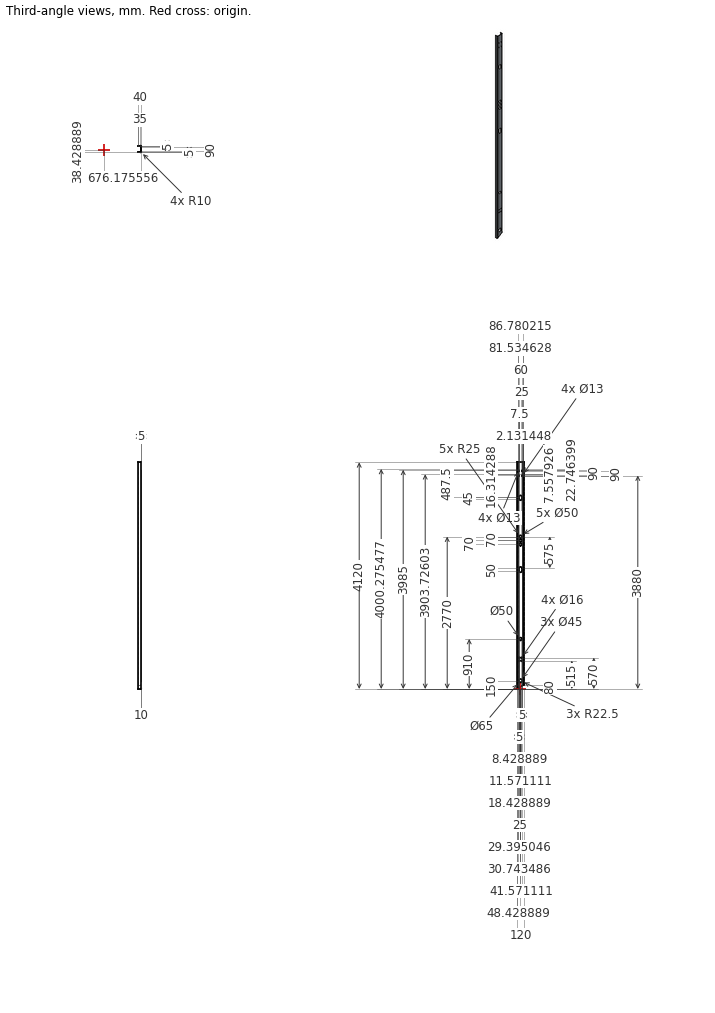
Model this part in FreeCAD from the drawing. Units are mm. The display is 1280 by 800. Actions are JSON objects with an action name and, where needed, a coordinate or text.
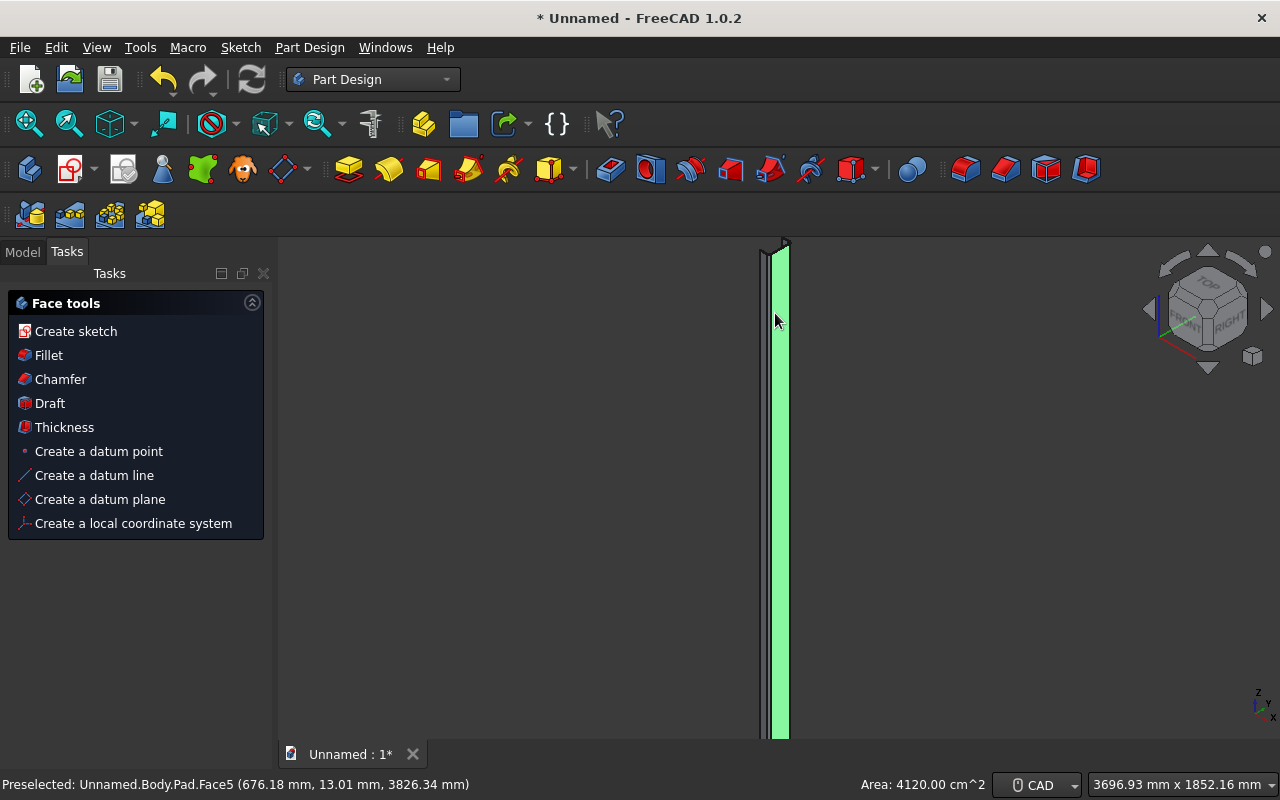
{"action": "left_click", "coordinate": [70, 170]}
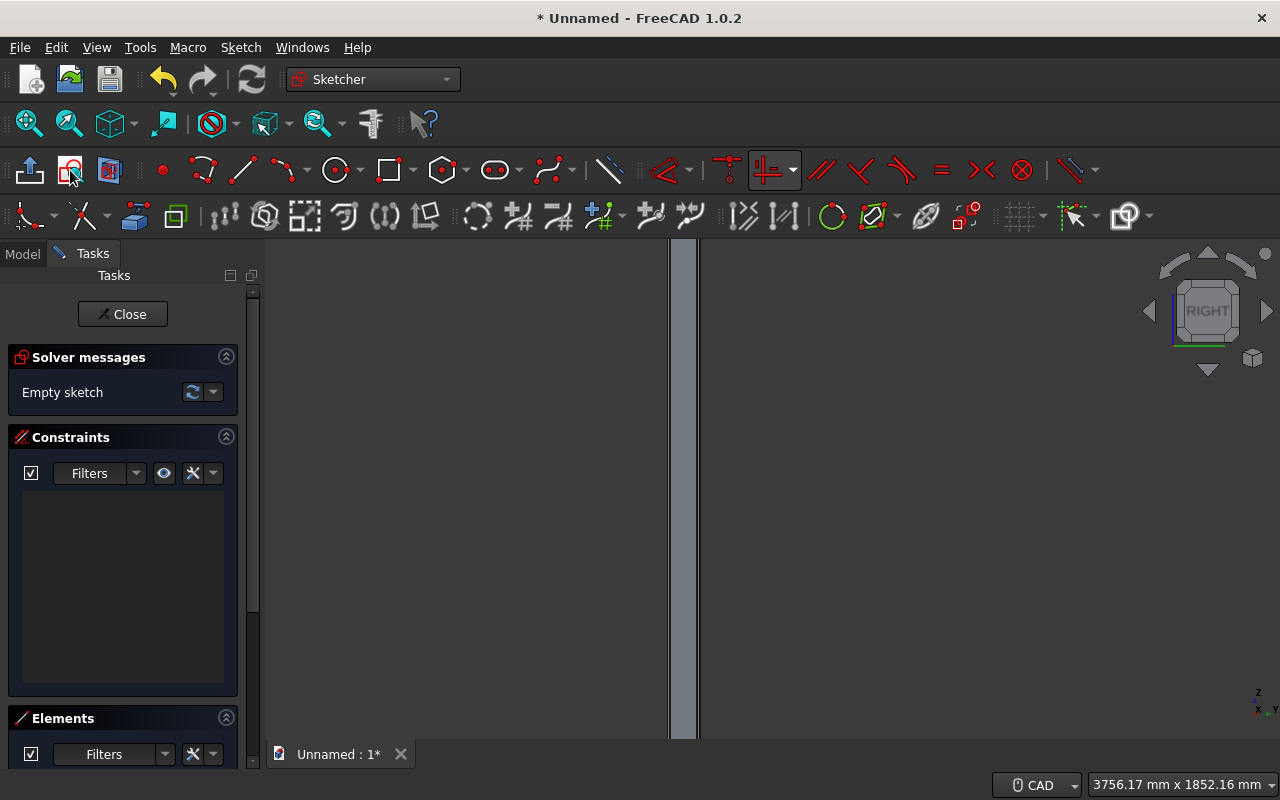
{"action": "scroll", "coordinate": [713, 406], "scroll_direction": "down", "scroll_amount": 6}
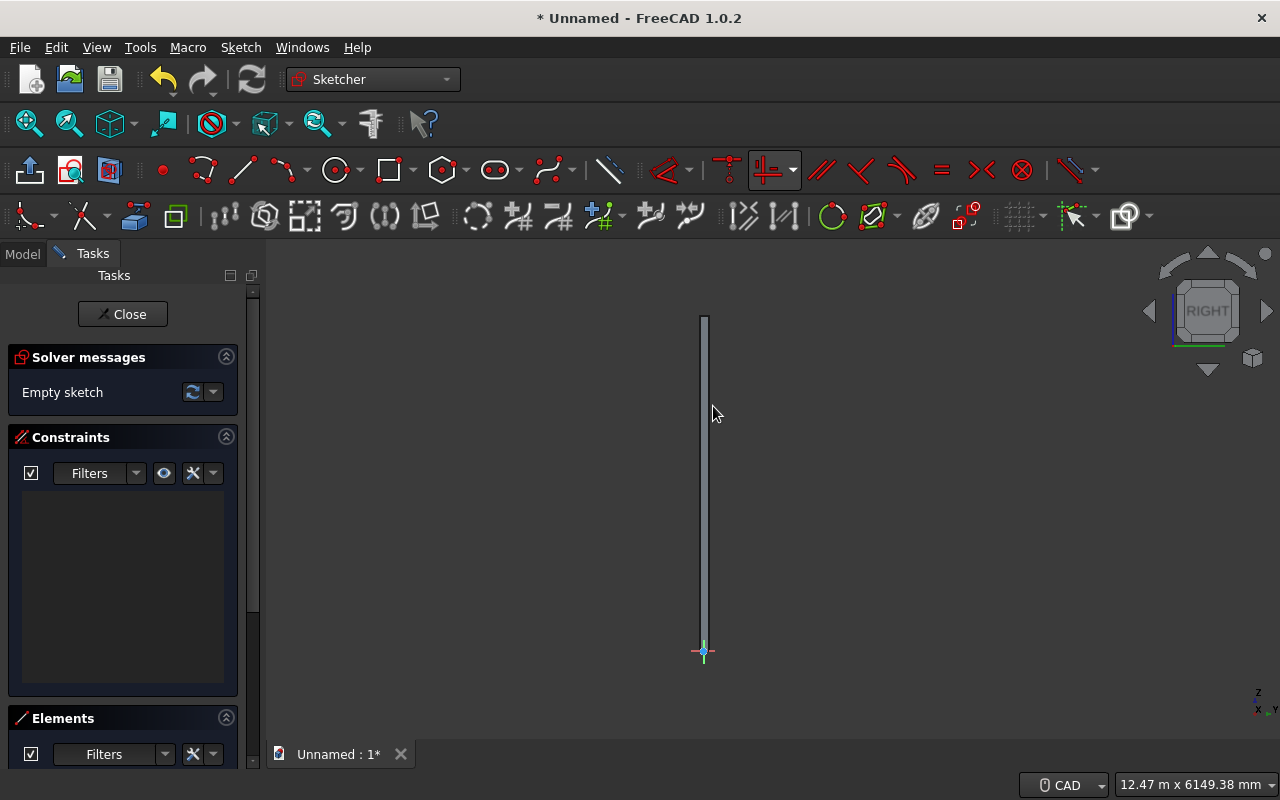
{"action": "left_click", "coordinate": [496, 170]}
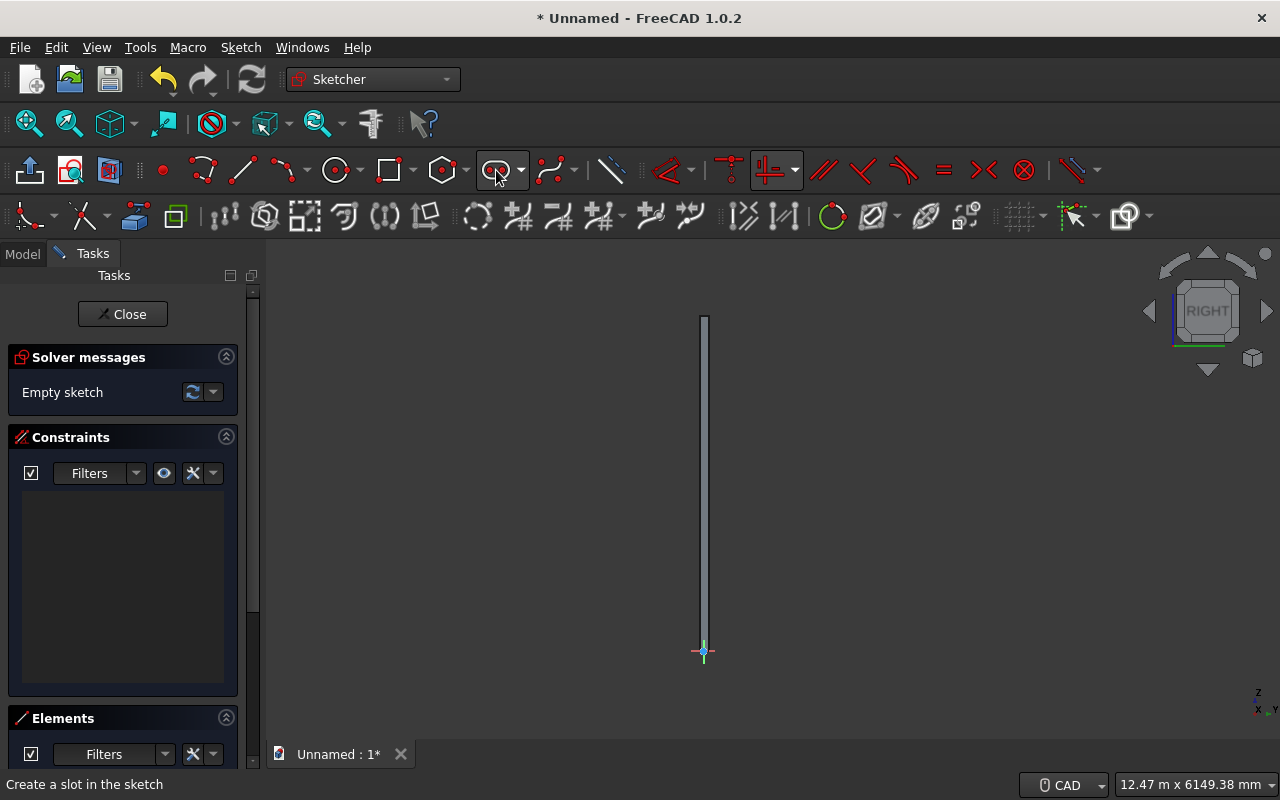
{"action": "scroll", "coordinate": [704, 370], "scroll_direction": "up", "scroll_amount": 15}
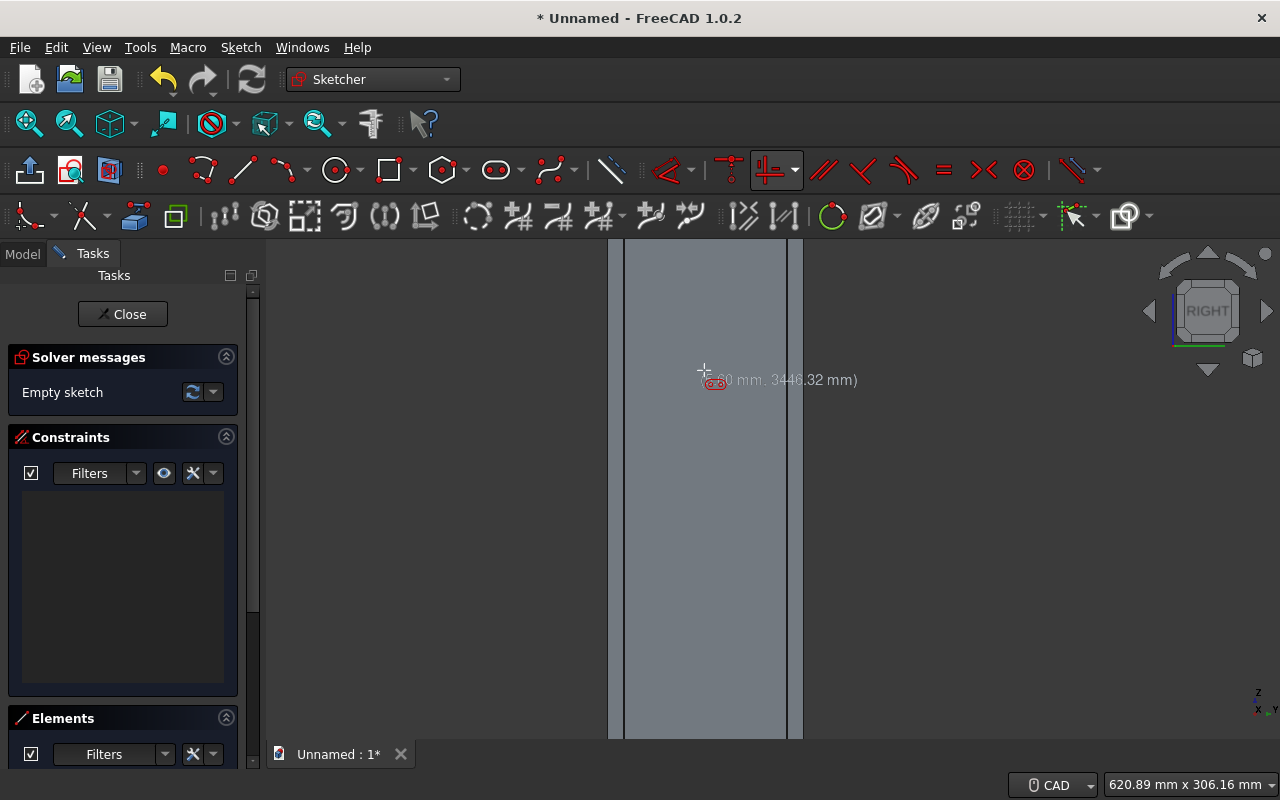
{"action": "left_click", "coordinate": [706, 375]}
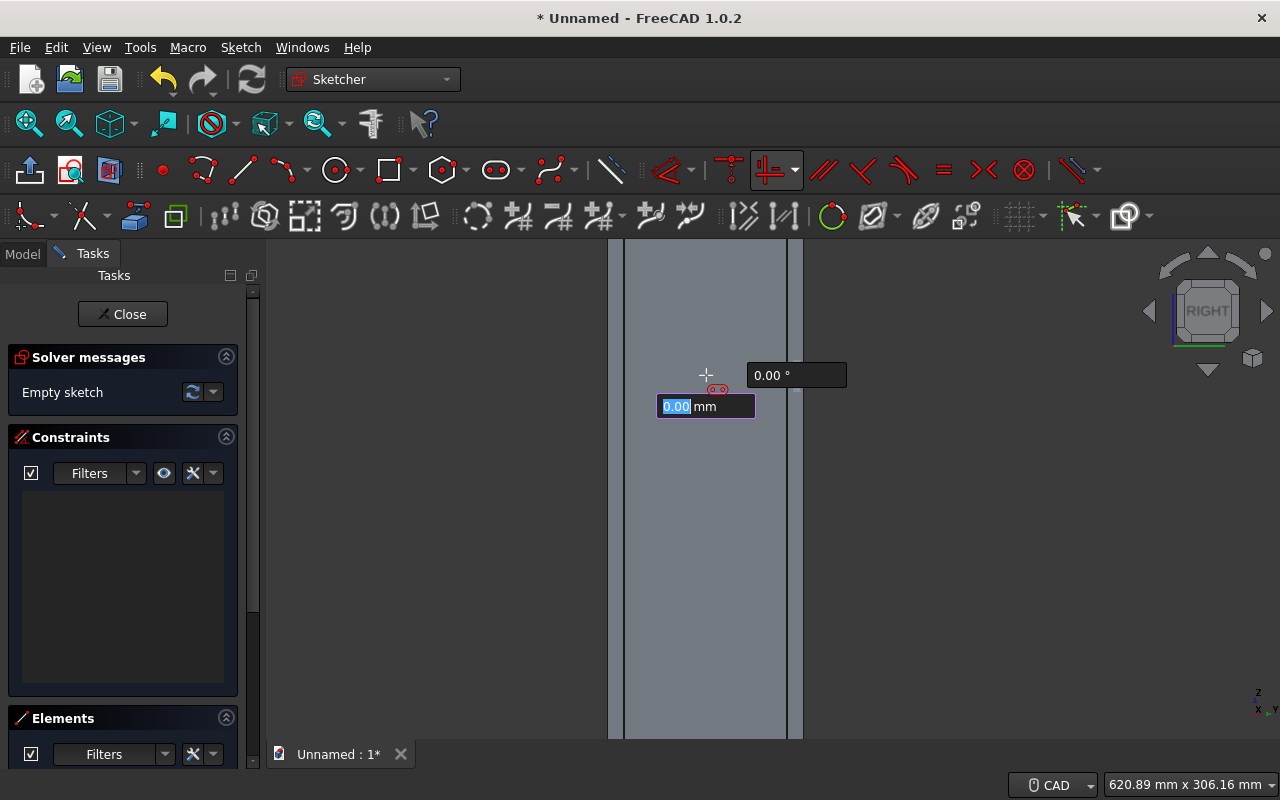
{"action": "left_click", "coordinate": [706, 301]}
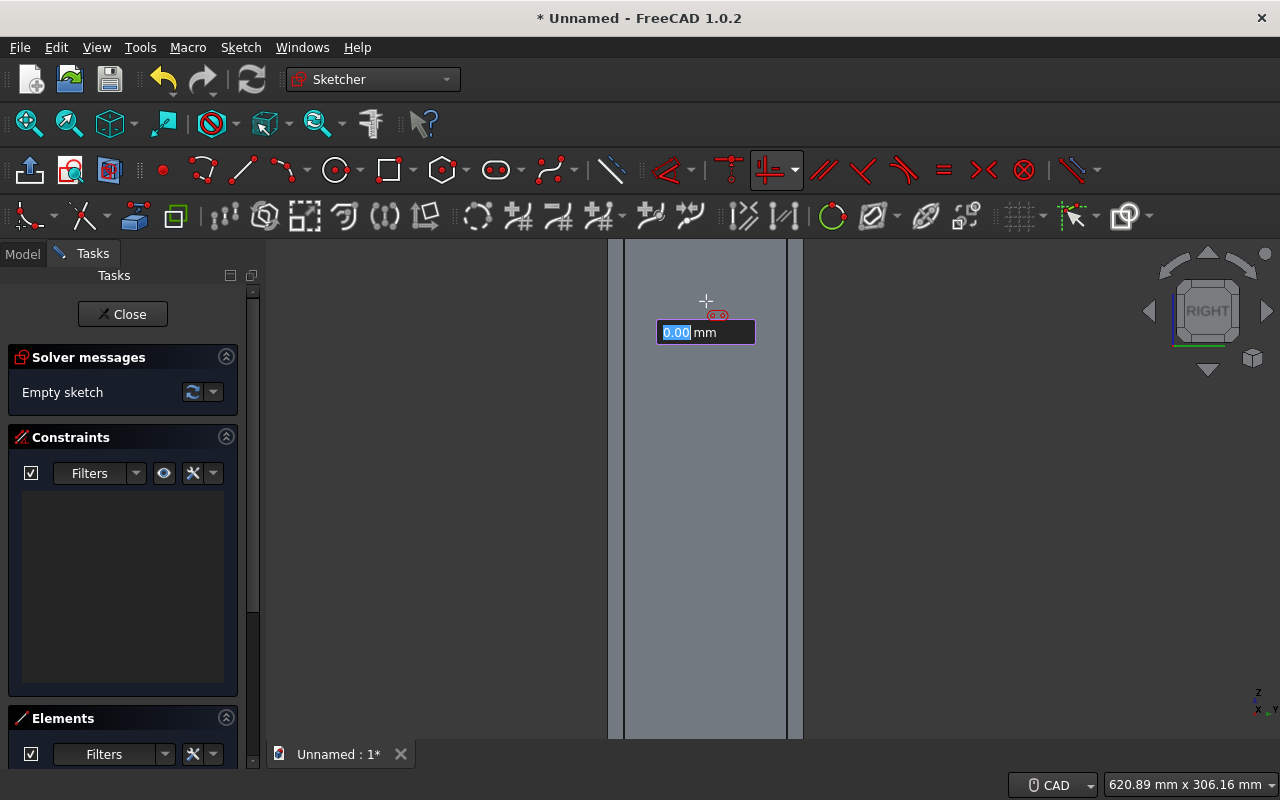
{"action": "left_click", "coordinate": [742, 338]}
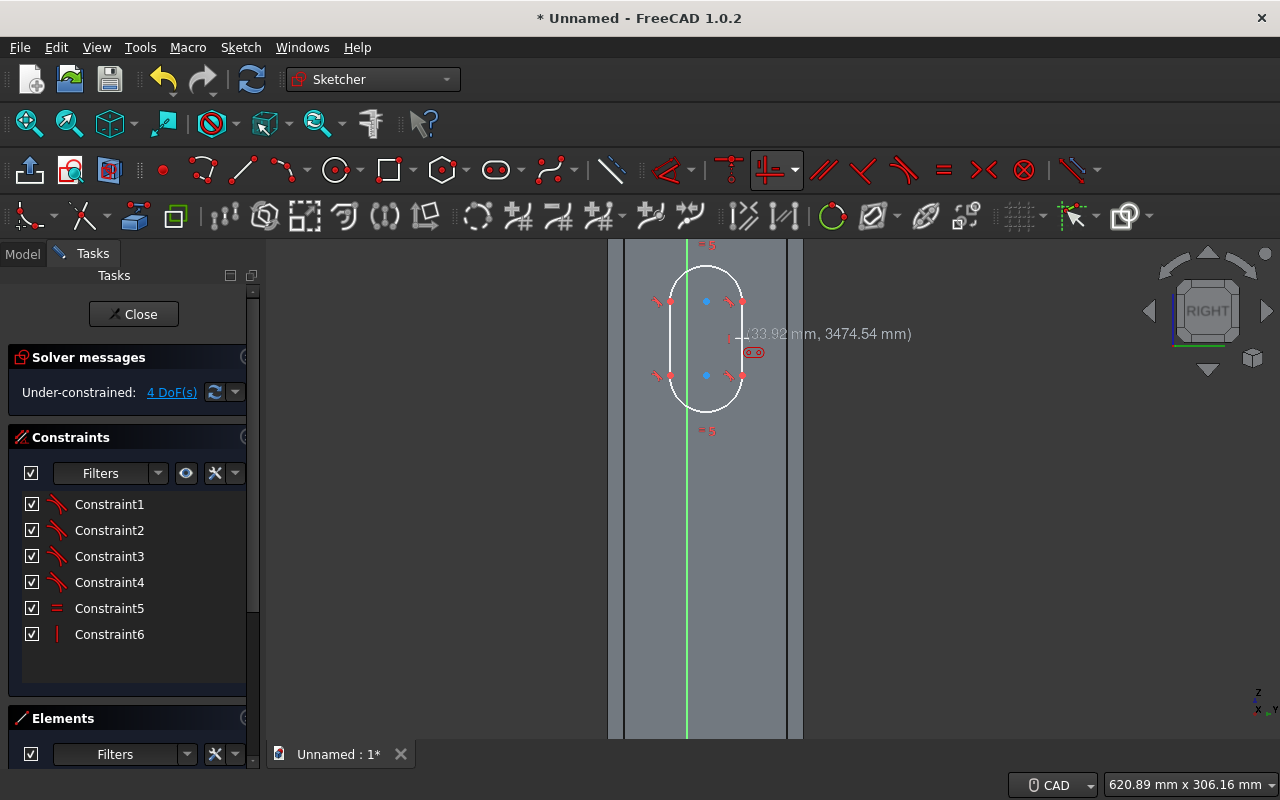
{"action": "scroll", "coordinate": [704, 370], "scroll_direction": "down", "scroll_amount": 15}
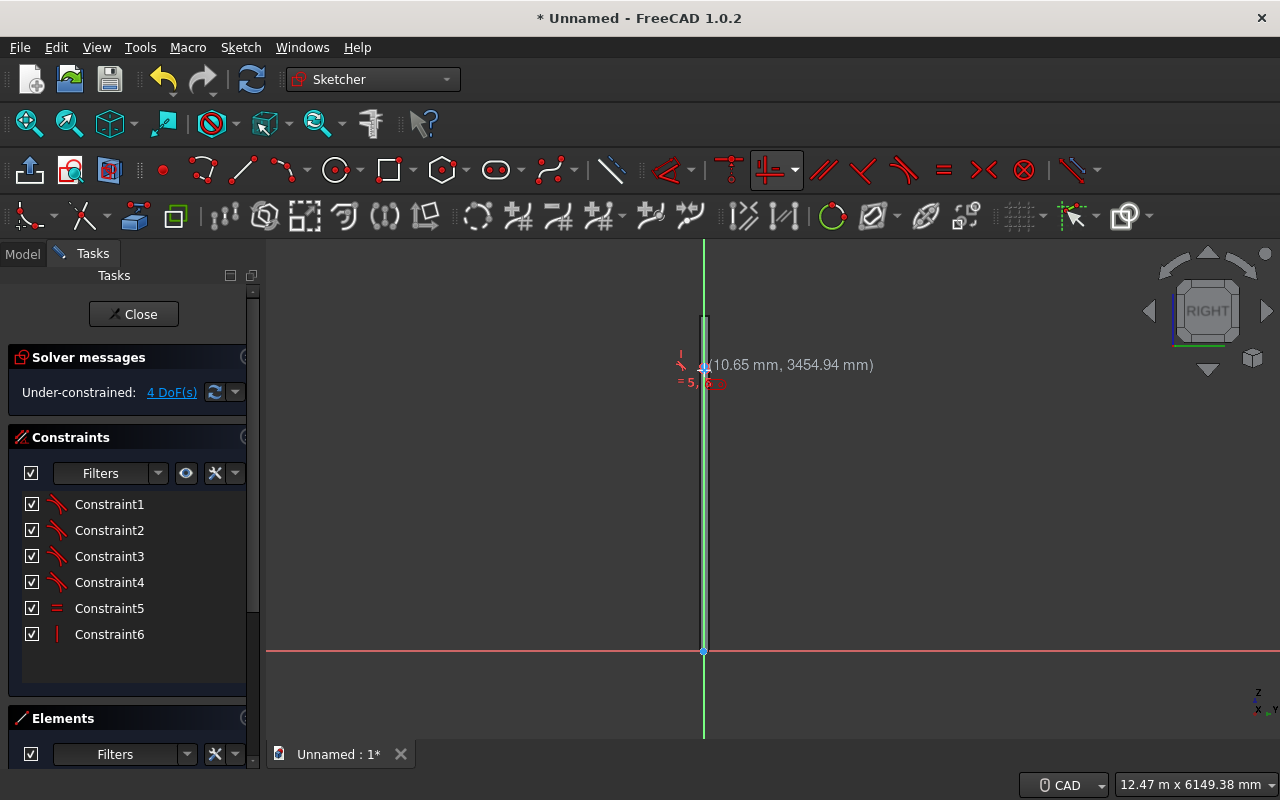
{"action": "scroll", "coordinate": [704, 477], "scroll_direction": "up", "scroll_amount": 15}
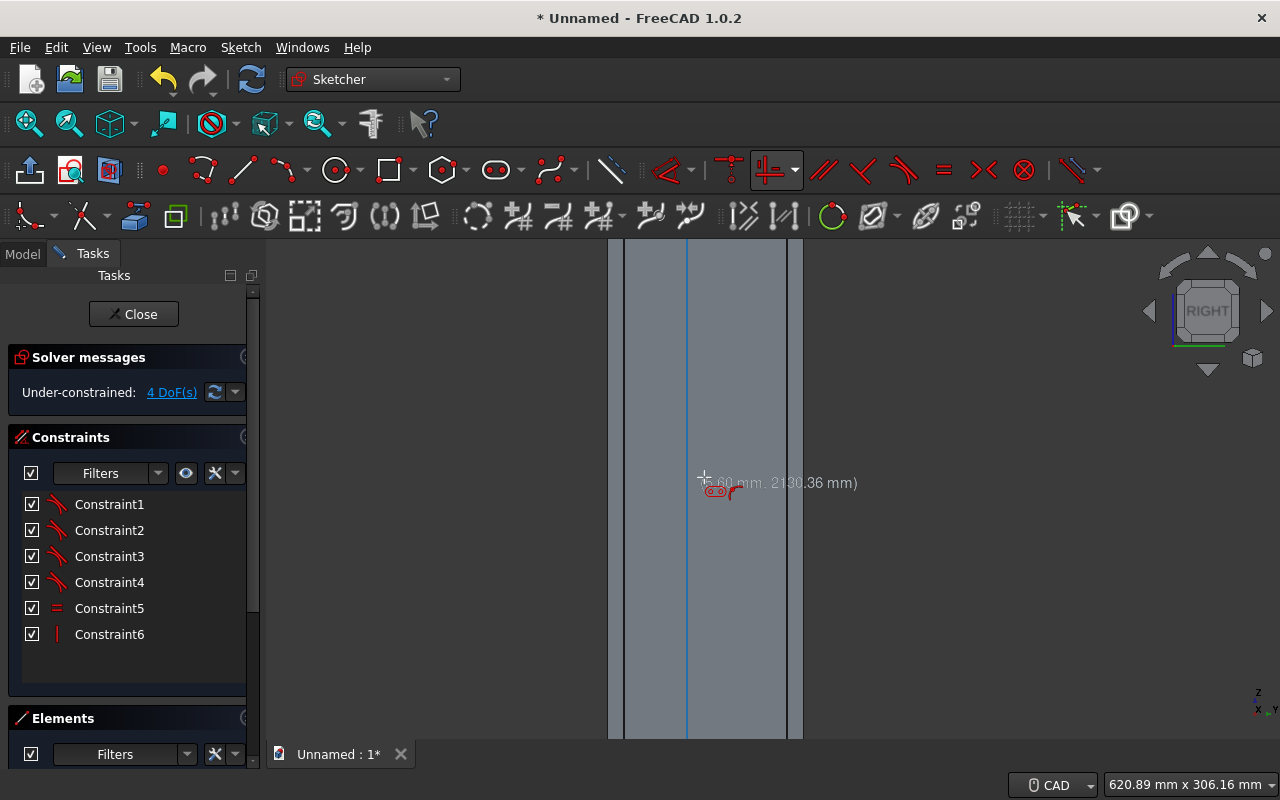
{"action": "left_click", "coordinate": [706, 464]}